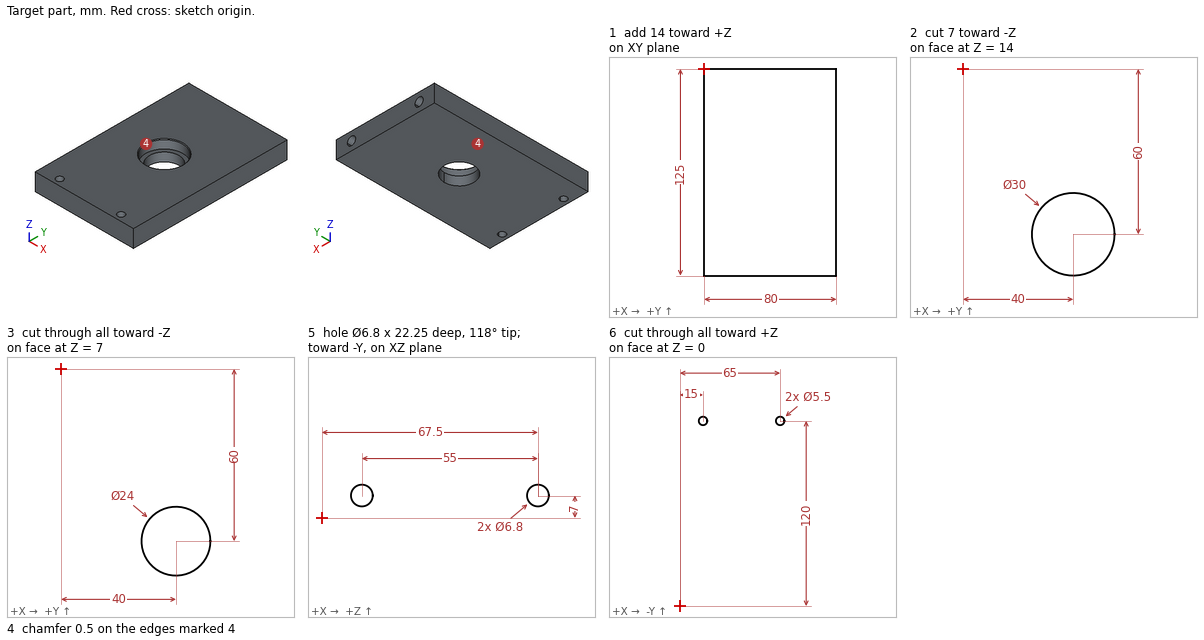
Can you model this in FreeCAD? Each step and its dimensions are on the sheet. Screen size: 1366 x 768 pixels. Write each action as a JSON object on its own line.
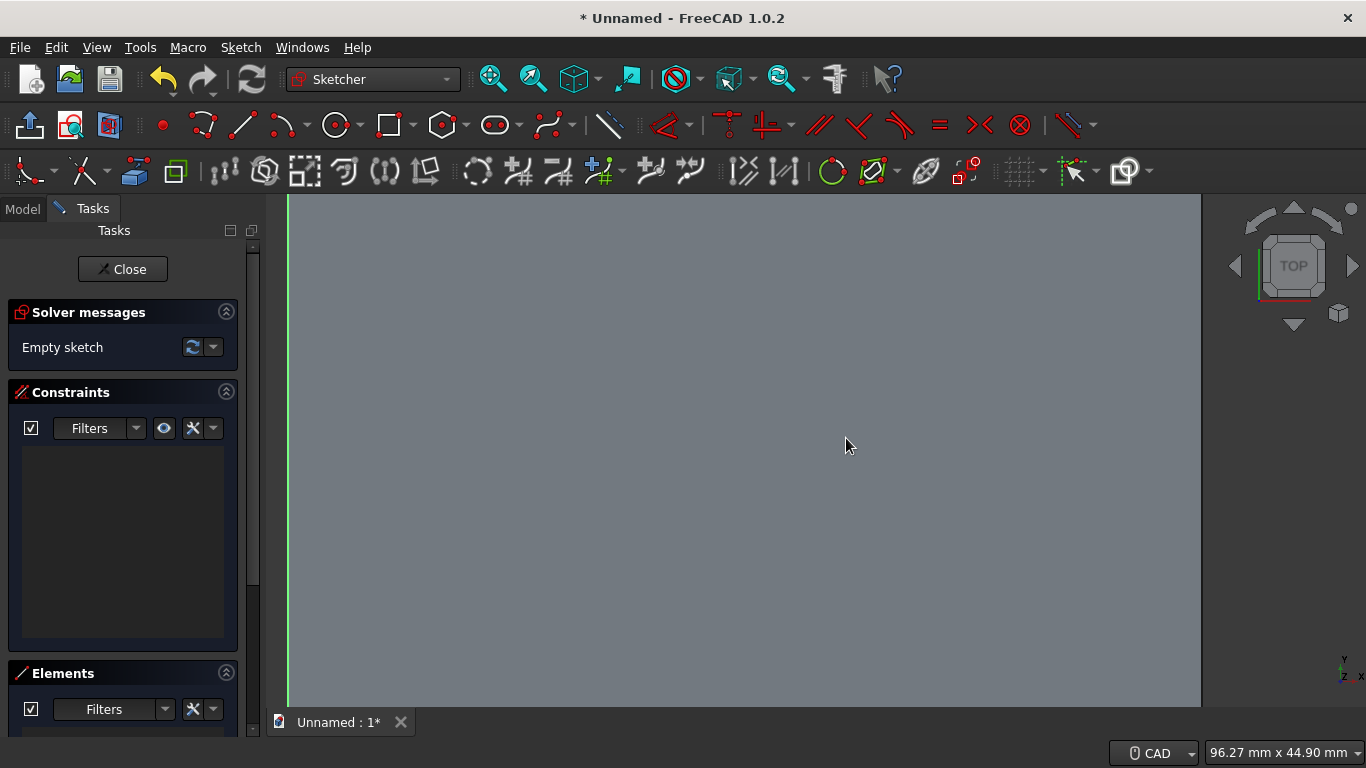
{"action": "left_click", "coordinate": [336, 126]}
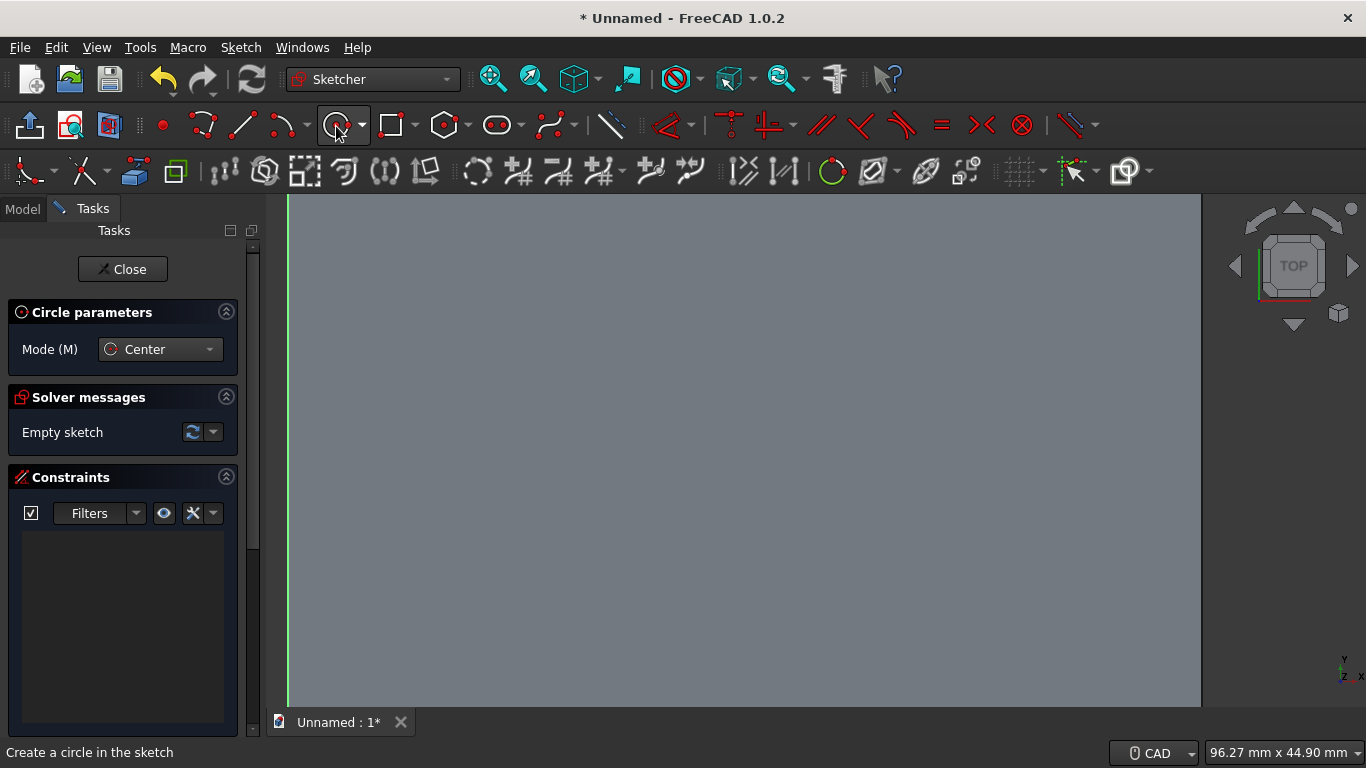
{"action": "left_click", "coordinate": [745, 450]}
{"action": "left_click", "coordinate": [866, 329]}
{"action": "key", "text": "Escape"}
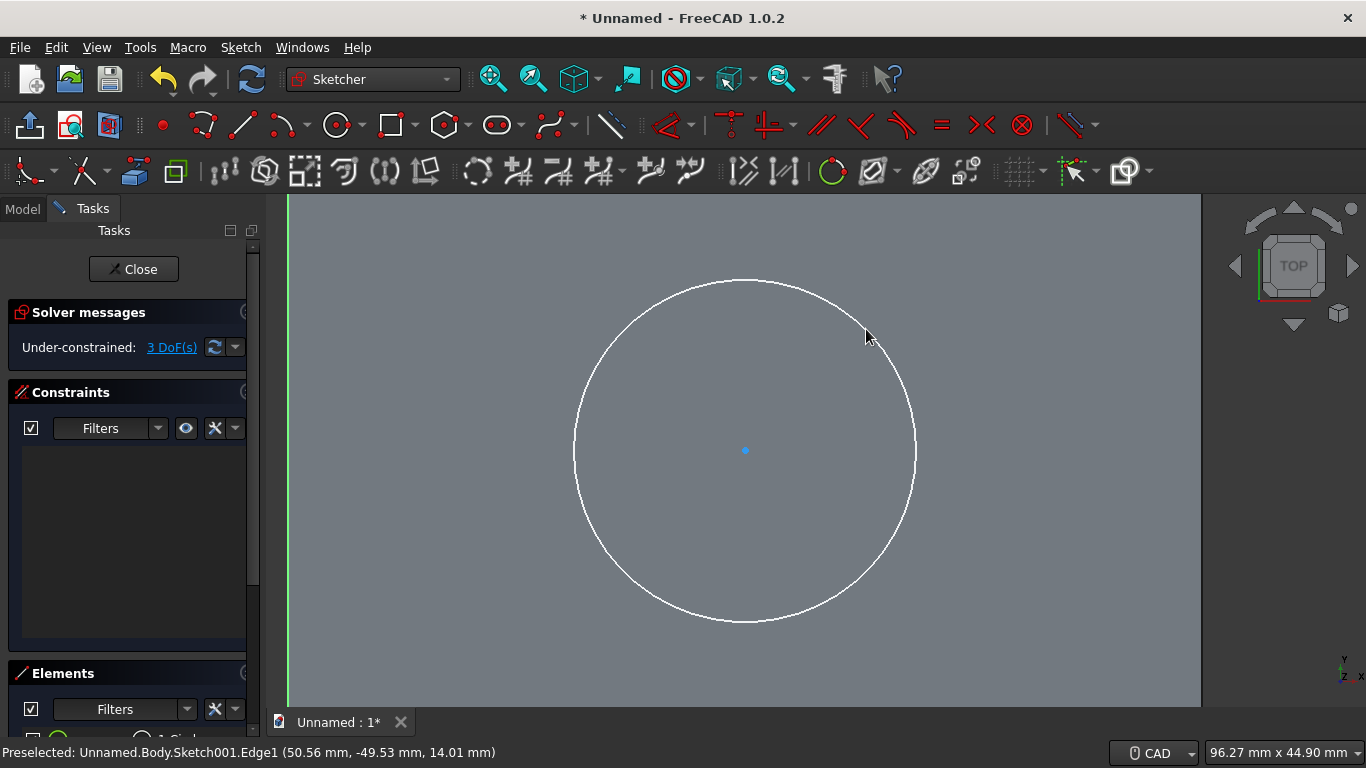
{"action": "left_click", "coordinate": [666, 126]}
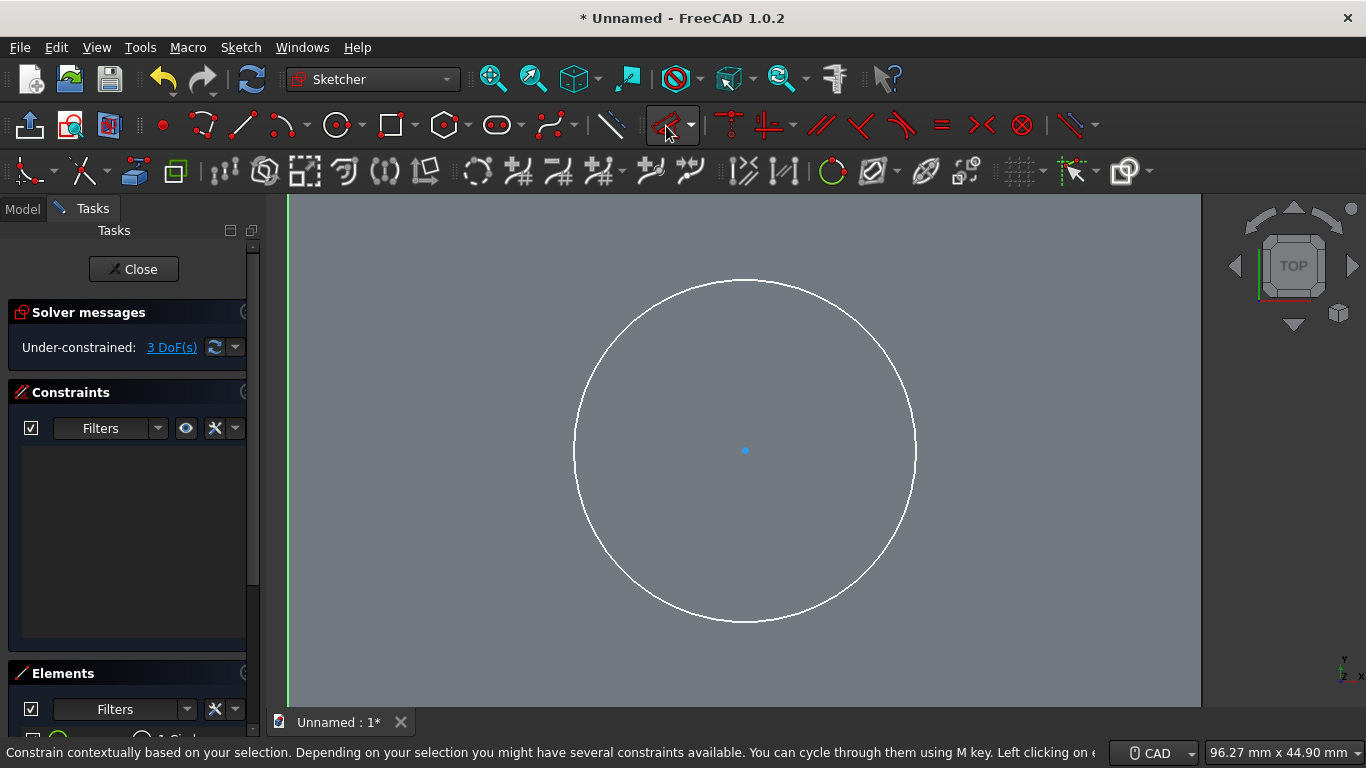
{"action": "left_click", "coordinate": [866, 330]}
{"action": "left_click", "coordinate": [889, 307]}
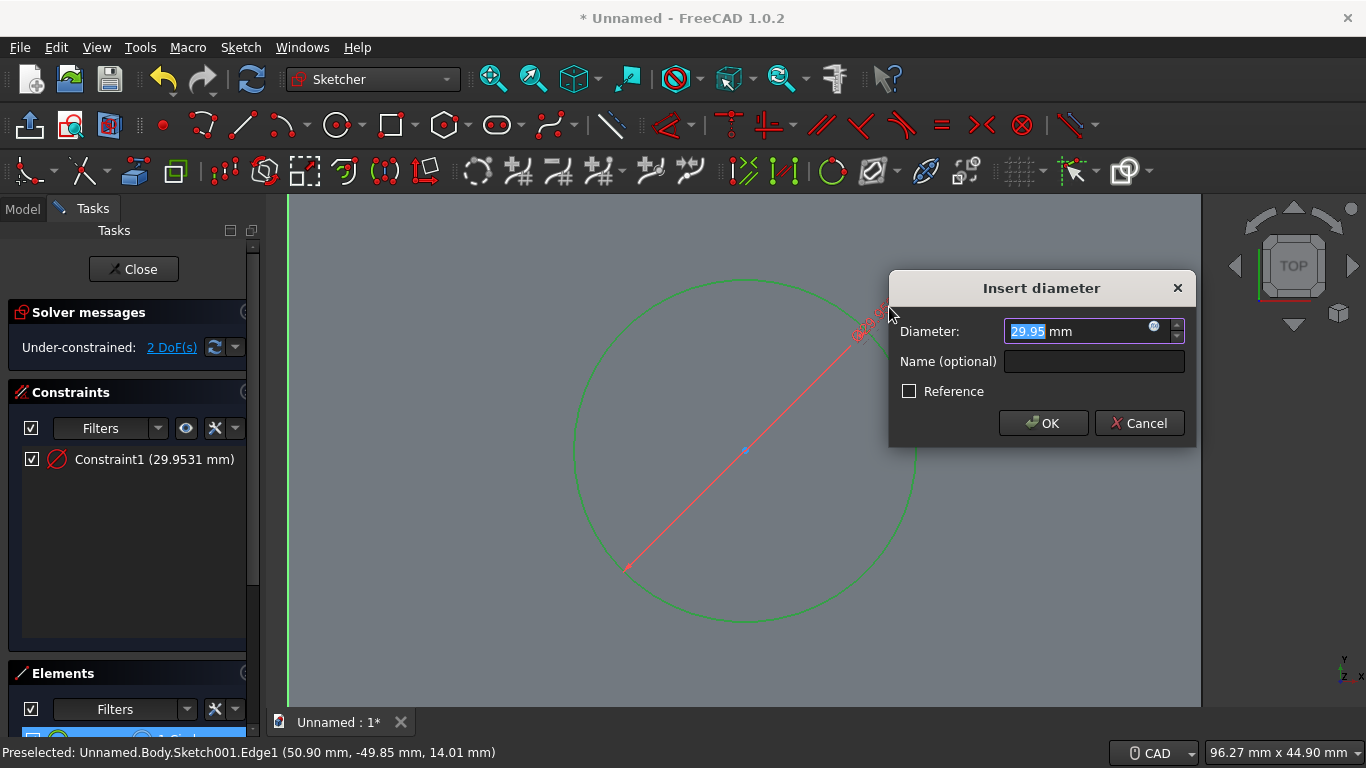
{"action": "type", "text": "30"}
{"action": "key", "text": "Return"}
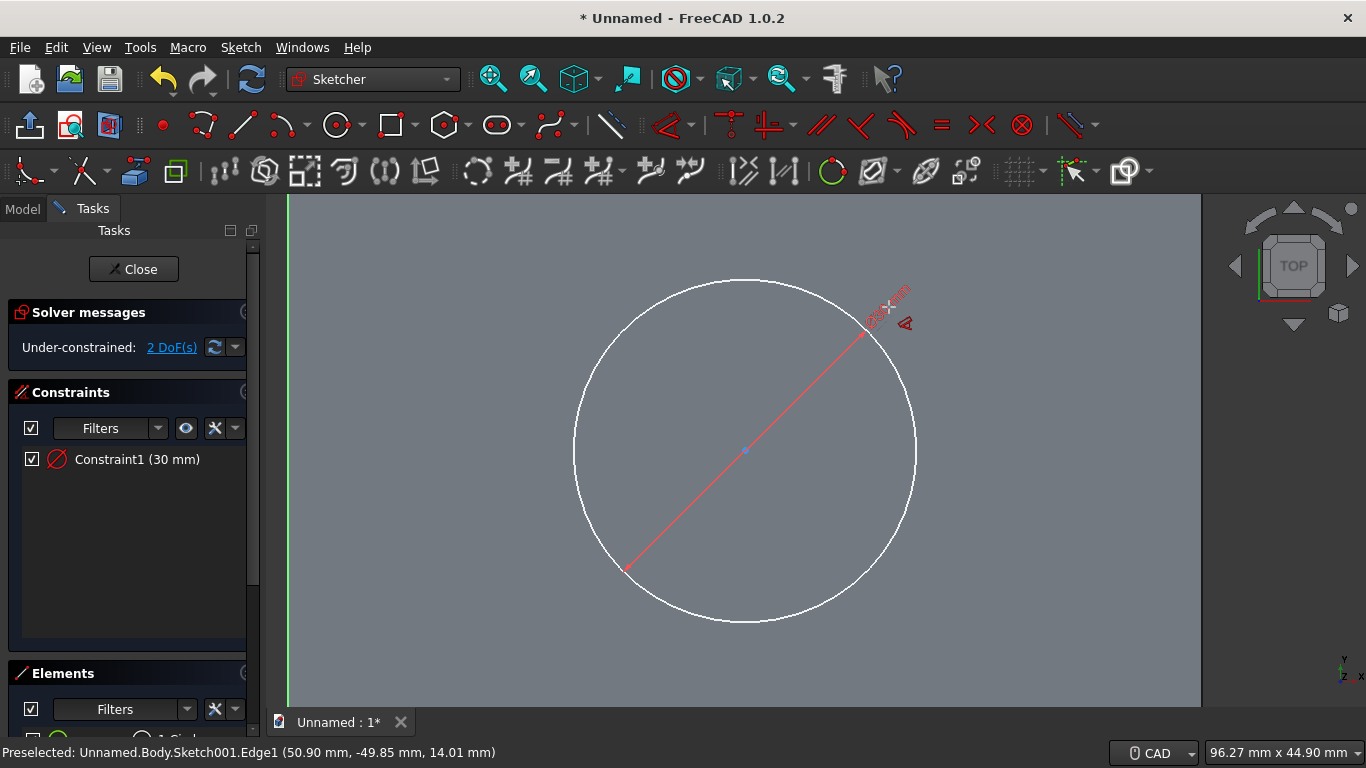
{"action": "left_click", "coordinate": [745, 451]}
{"action": "left_click", "coordinate": [519, 485]}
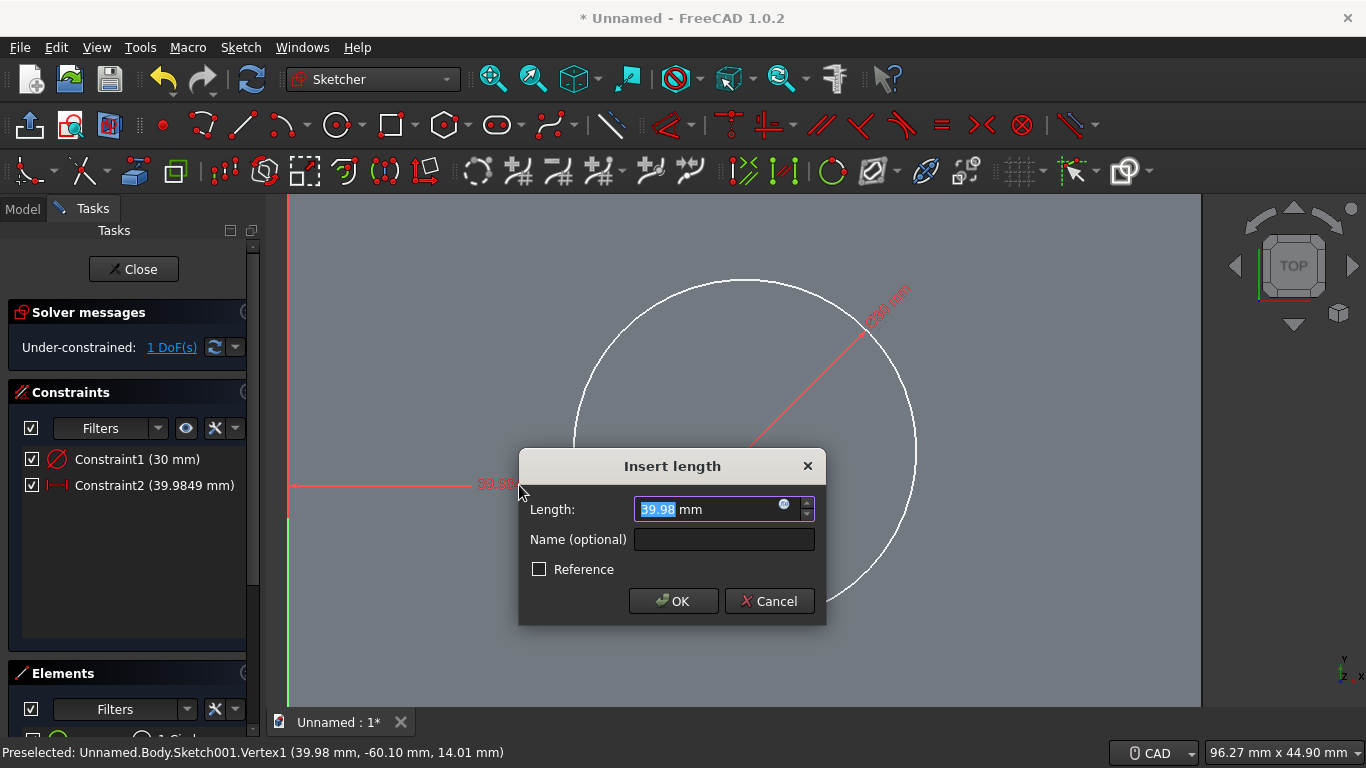
{"action": "type", "text": "40"}
{"action": "key", "text": "Return"}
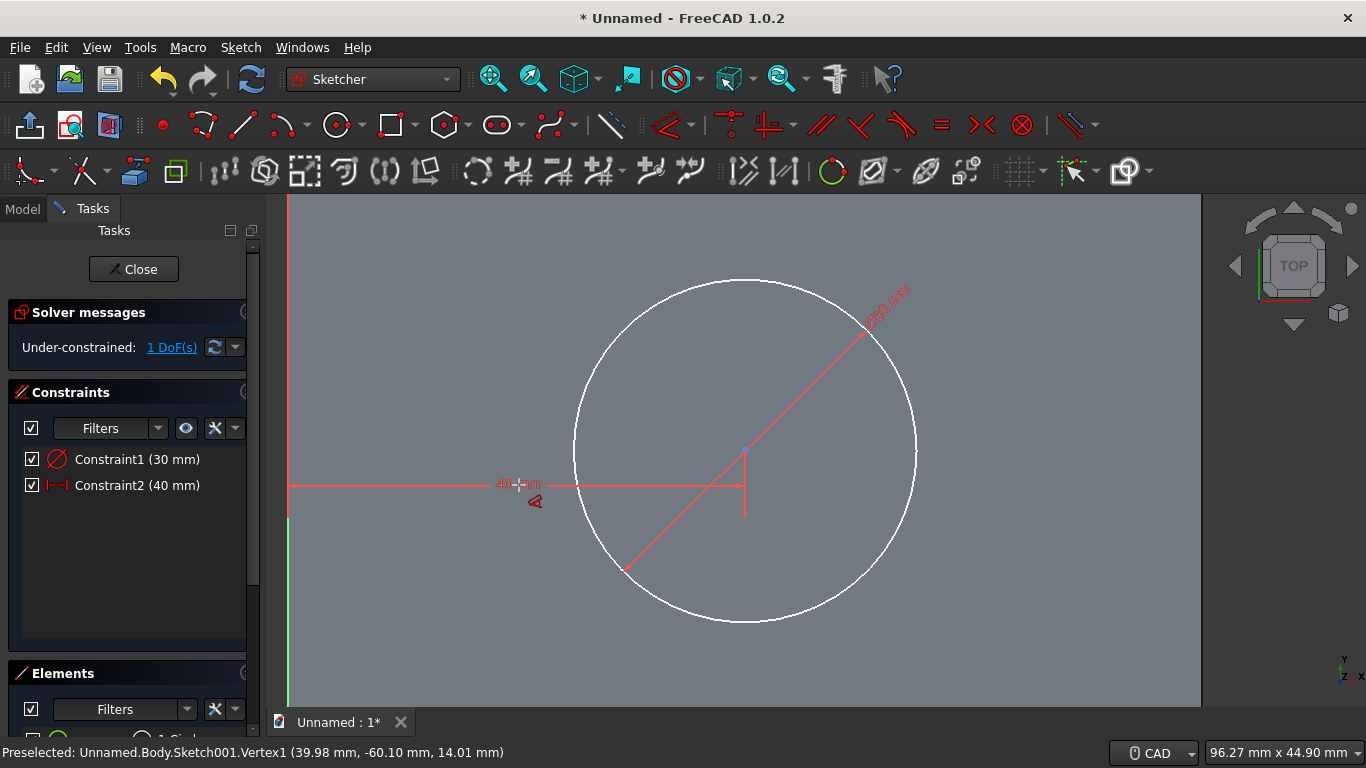
{"action": "left_click", "coordinate": [745, 451]}
{"action": "left_click", "coordinate": [779, 336]}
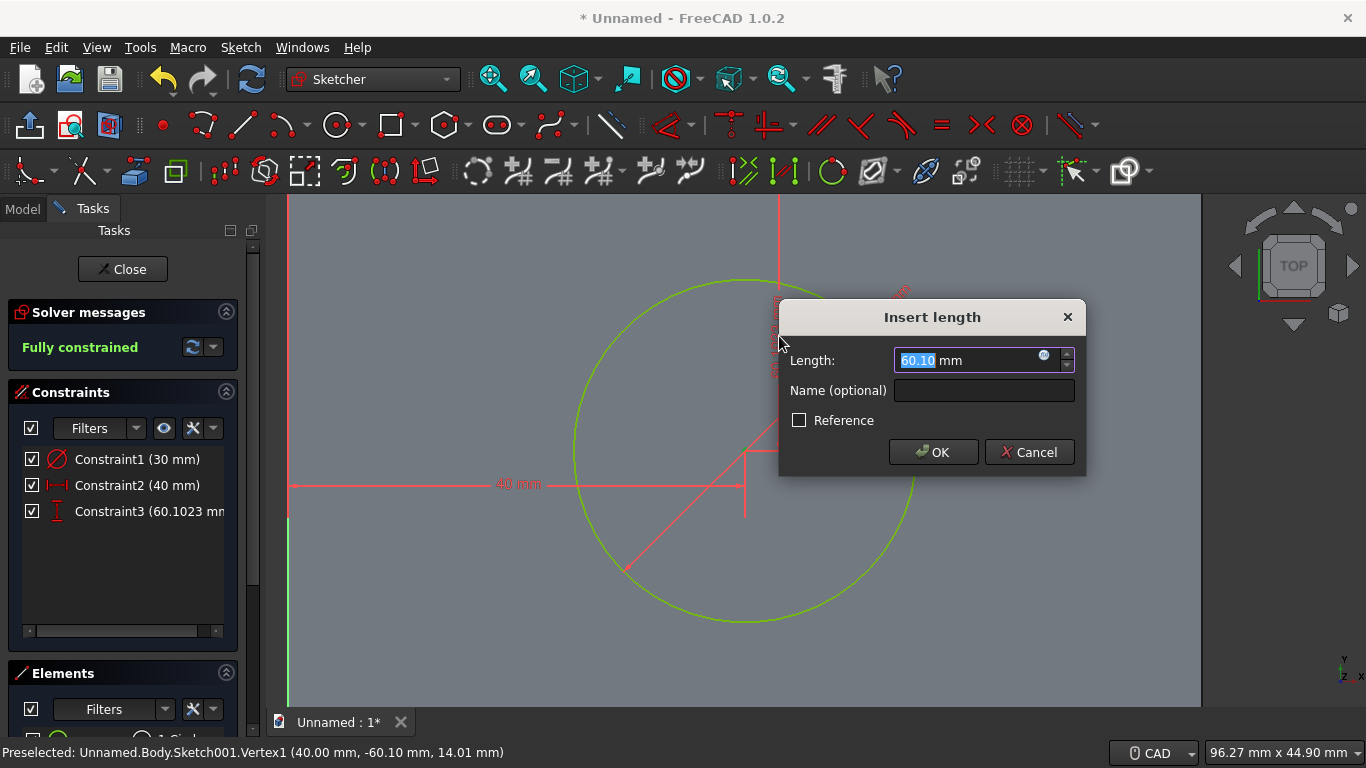
{"action": "type", "text": "60"}
{"action": "key", "text": "Return"}
{"action": "key", "text": "Escape"}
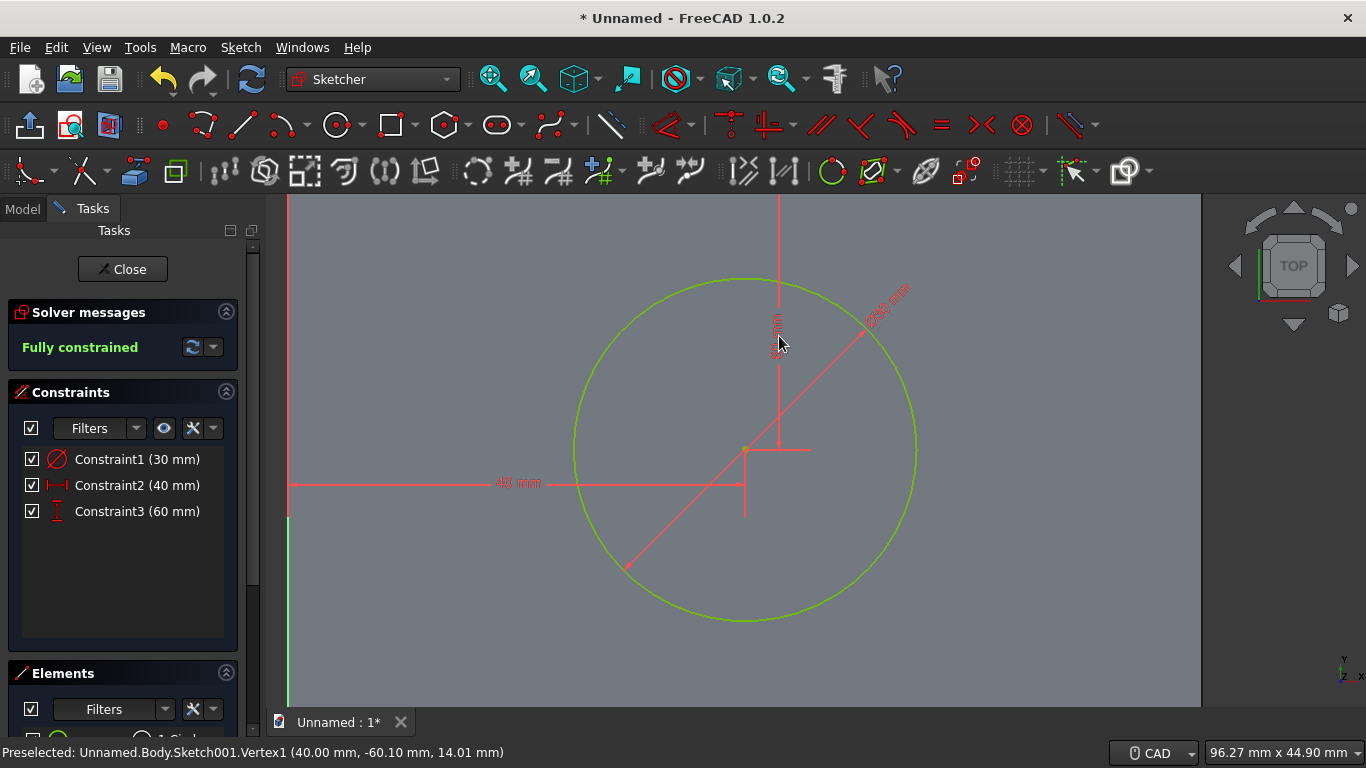
{"action": "left_click", "coordinate": [123, 269]}